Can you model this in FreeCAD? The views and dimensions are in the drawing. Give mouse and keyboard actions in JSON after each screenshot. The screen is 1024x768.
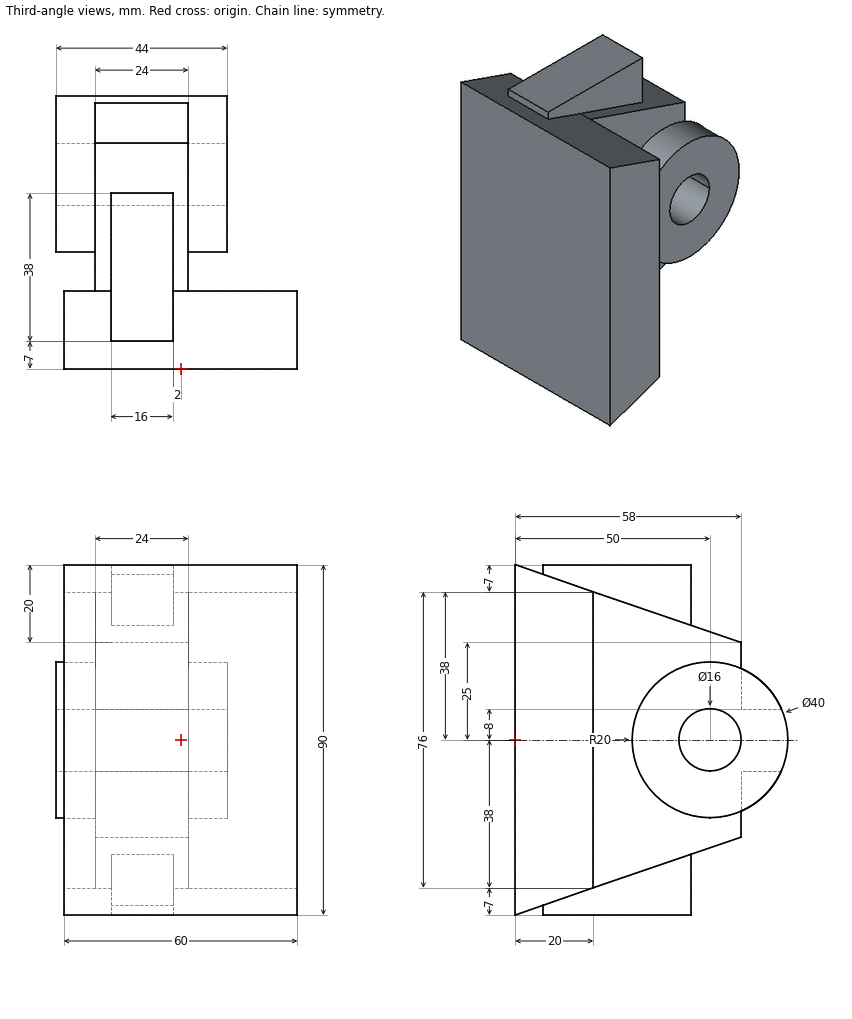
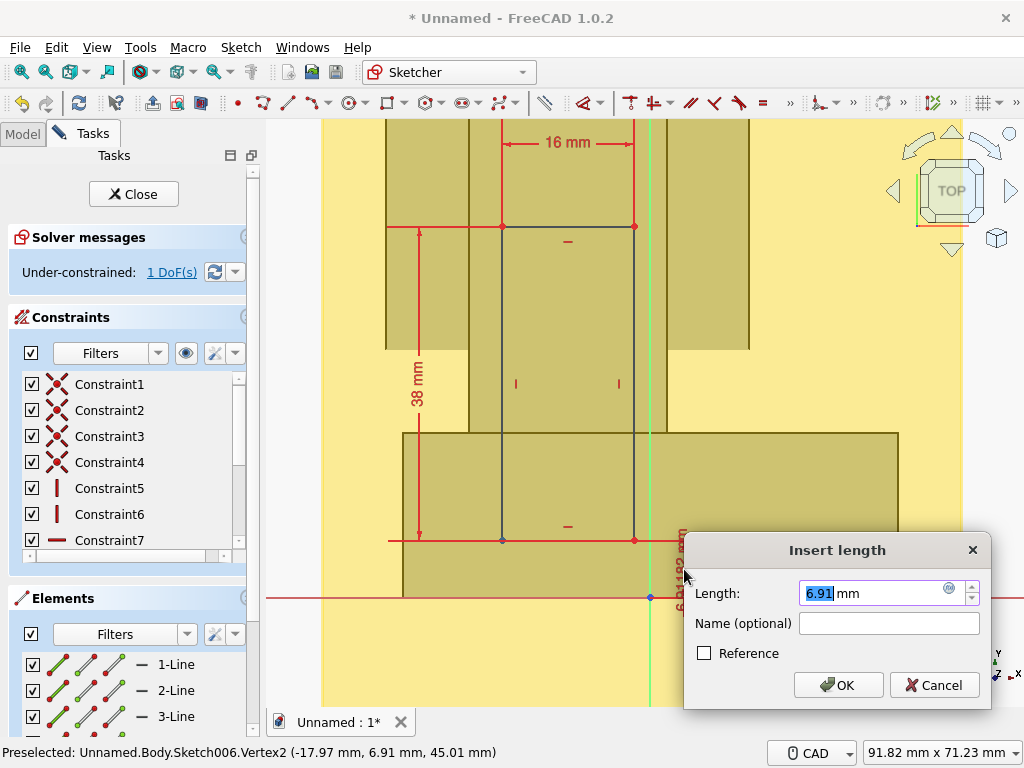
{"action": "type", "text": "7"}
{"action": "key", "text": "Return"}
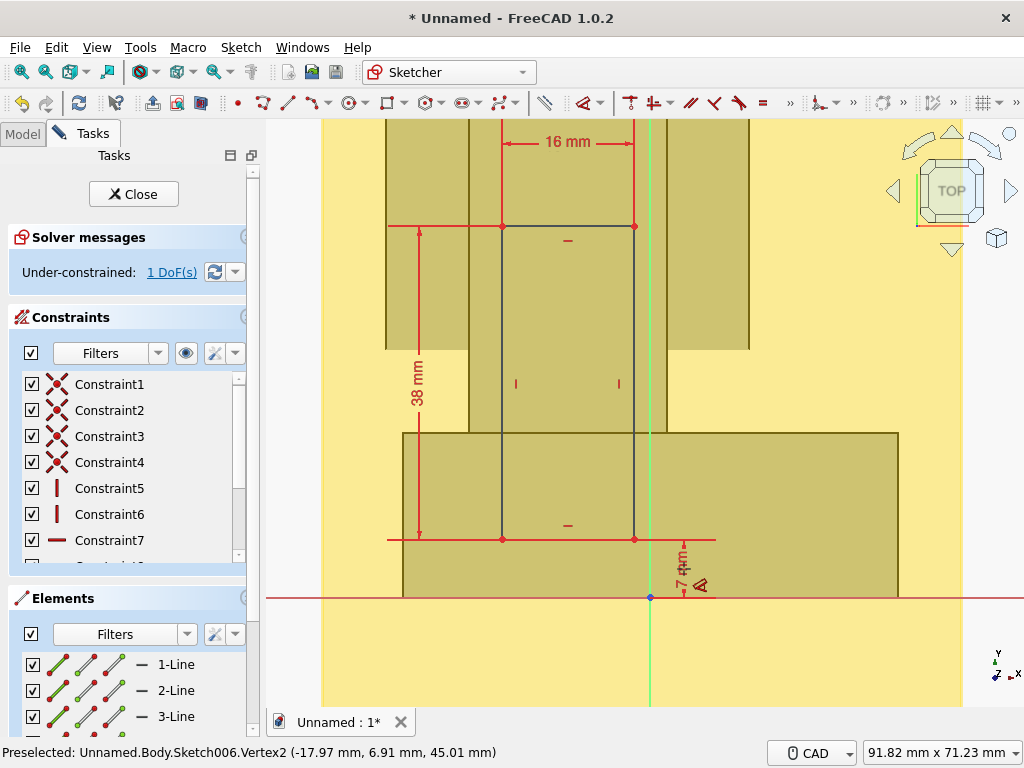
{"action": "scroll", "coordinate": [634, 540], "scroll_direction": "up", "scroll_amount": 5}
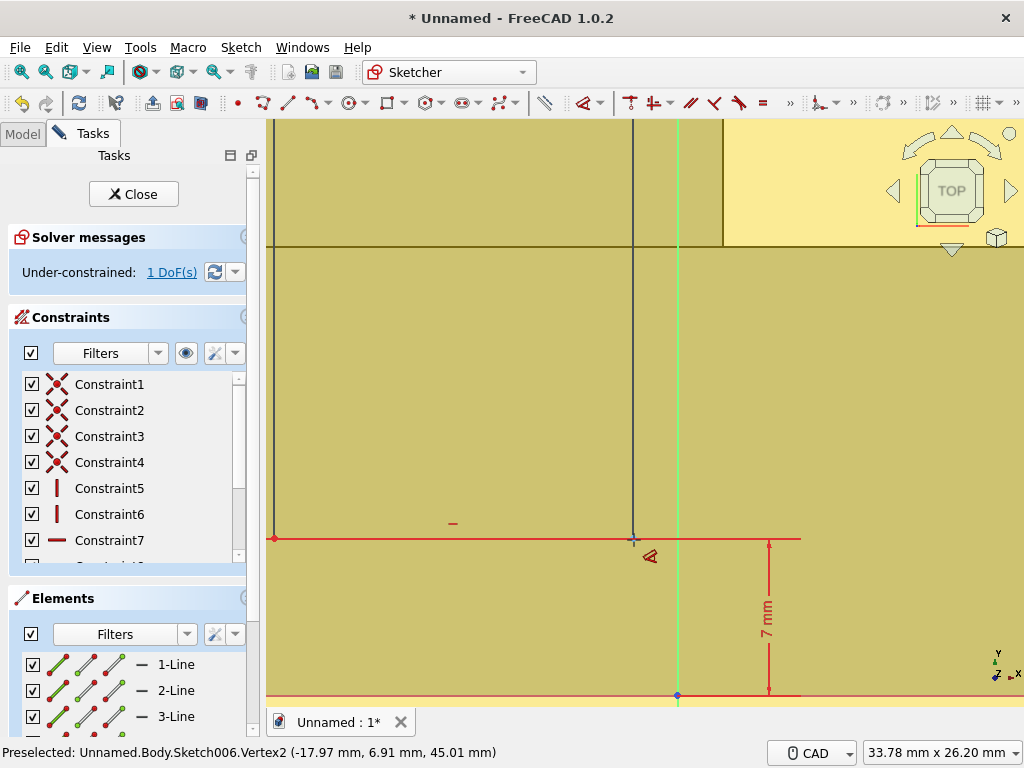
{"action": "left_click", "coordinate": [633, 539]}
{"action": "left_click", "coordinate": [656, 505]}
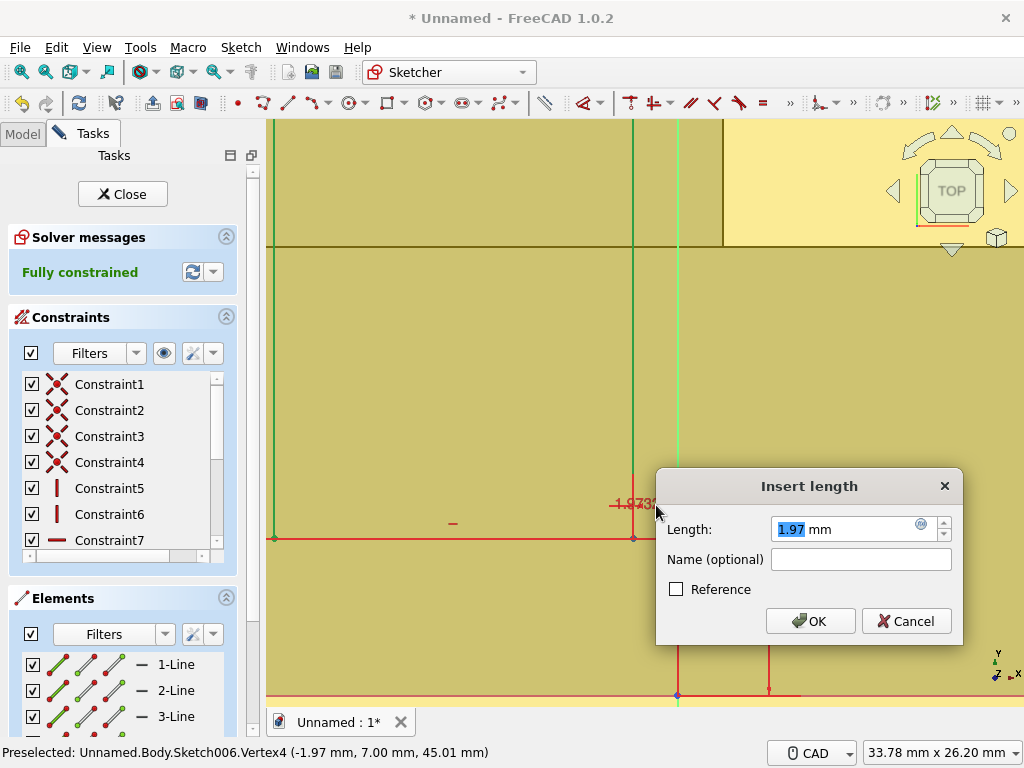
{"action": "type", "text": "2"}
{"action": "key", "text": "Return"}
{"action": "key", "text": "Escape"}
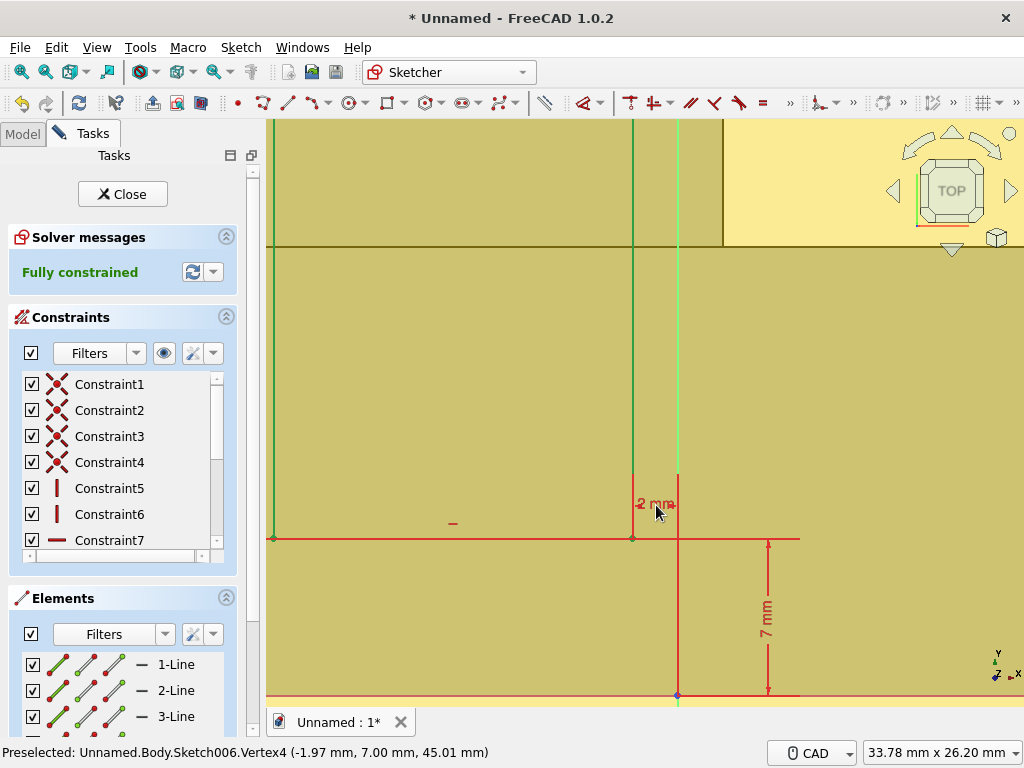
{"action": "left_click", "coordinate": [123, 194]}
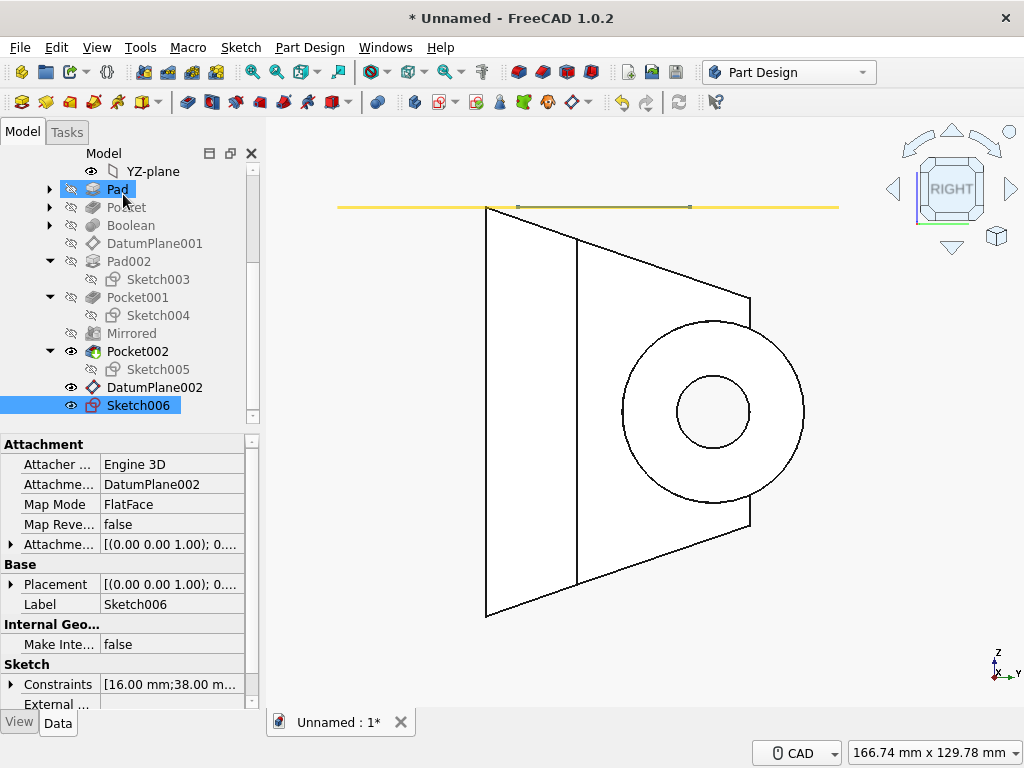
{"action": "left_click", "coordinate": [22, 102]}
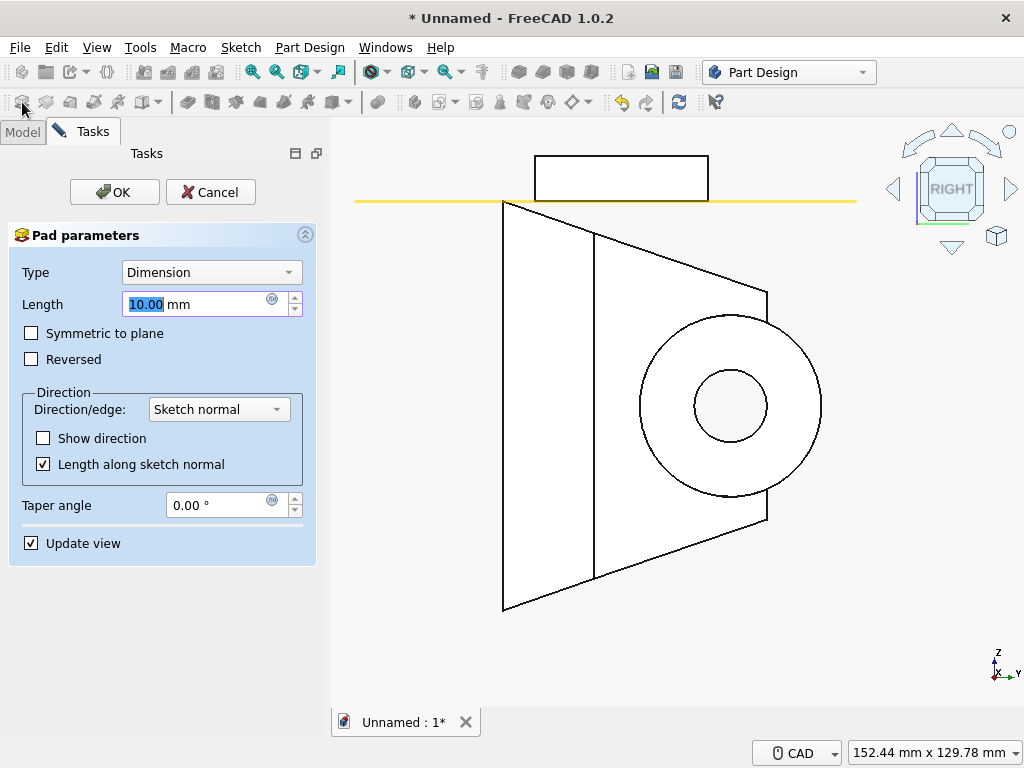
{"action": "type", "text": "20"}
{"action": "key", "text": "Tab"}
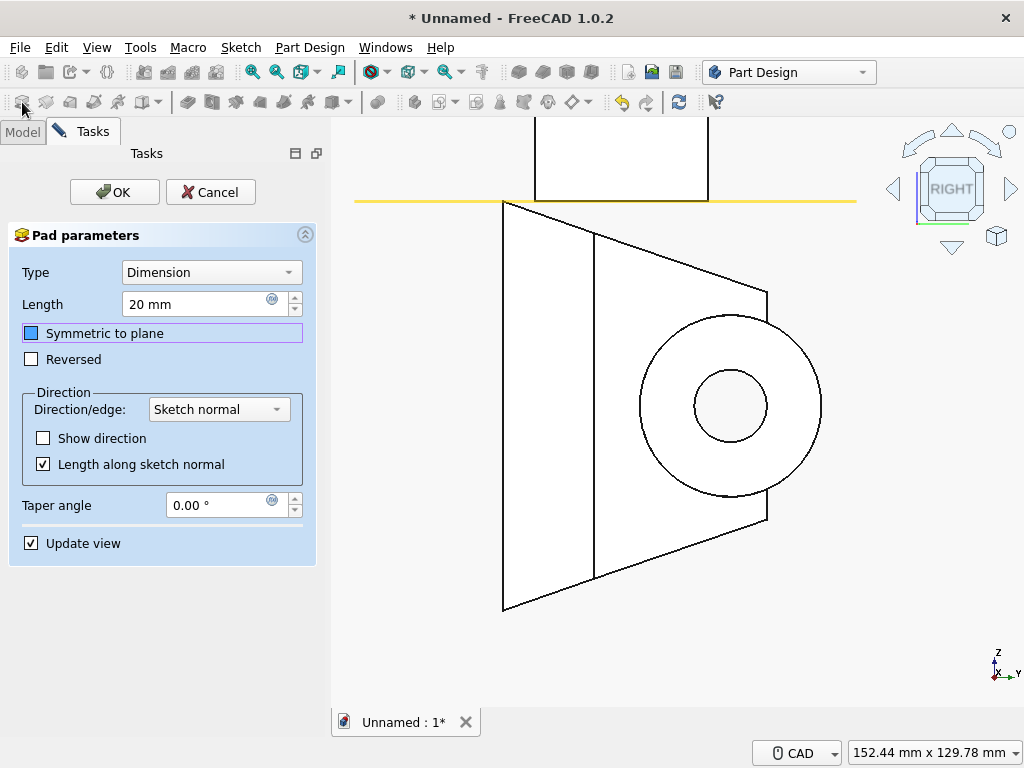
{"action": "left_click", "coordinate": [30, 359]}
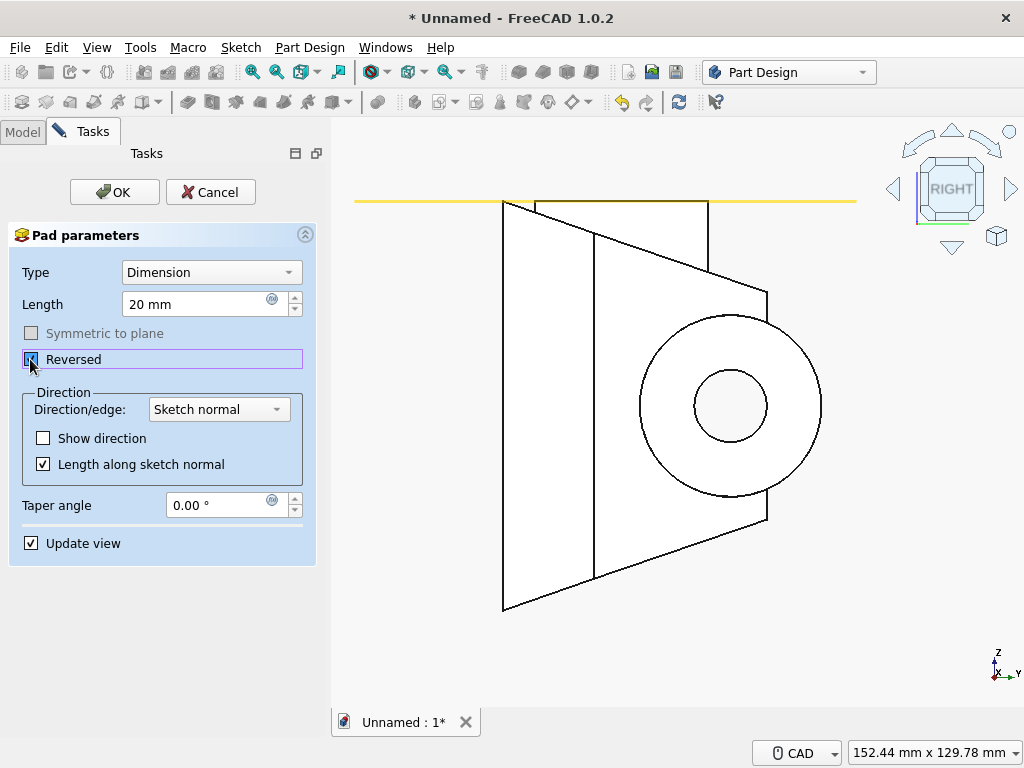
{"action": "left_click", "coordinate": [115, 192]}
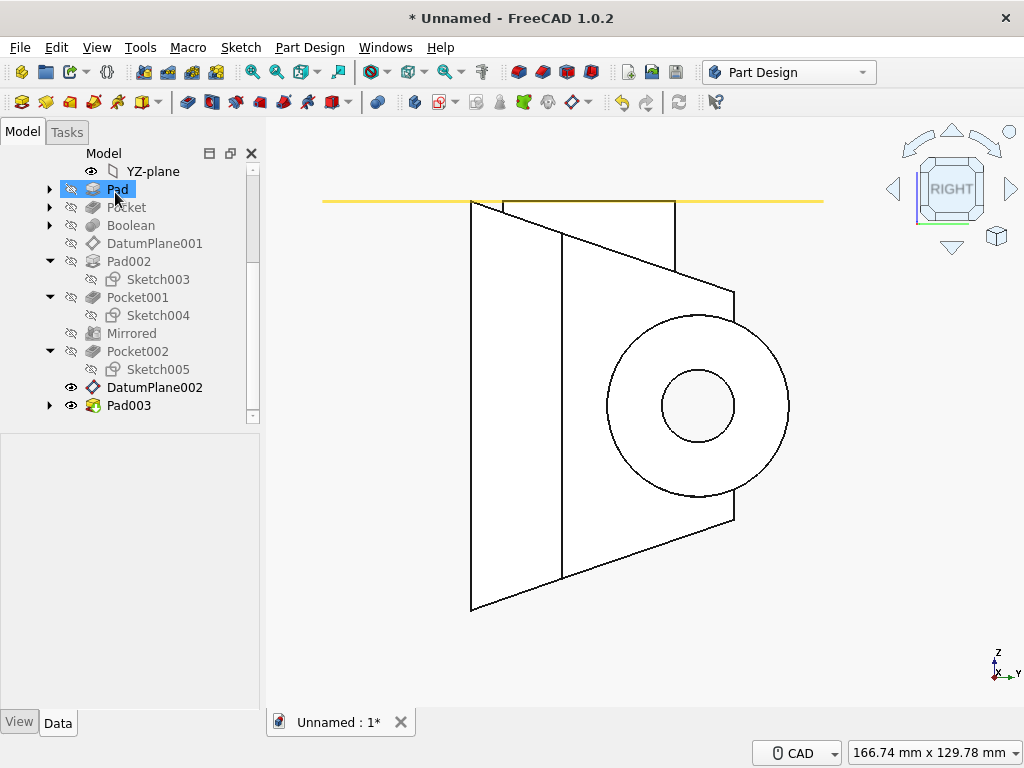
{"action": "left_click", "coordinate": [116, 387]}
{"action": "key", "text": "space"}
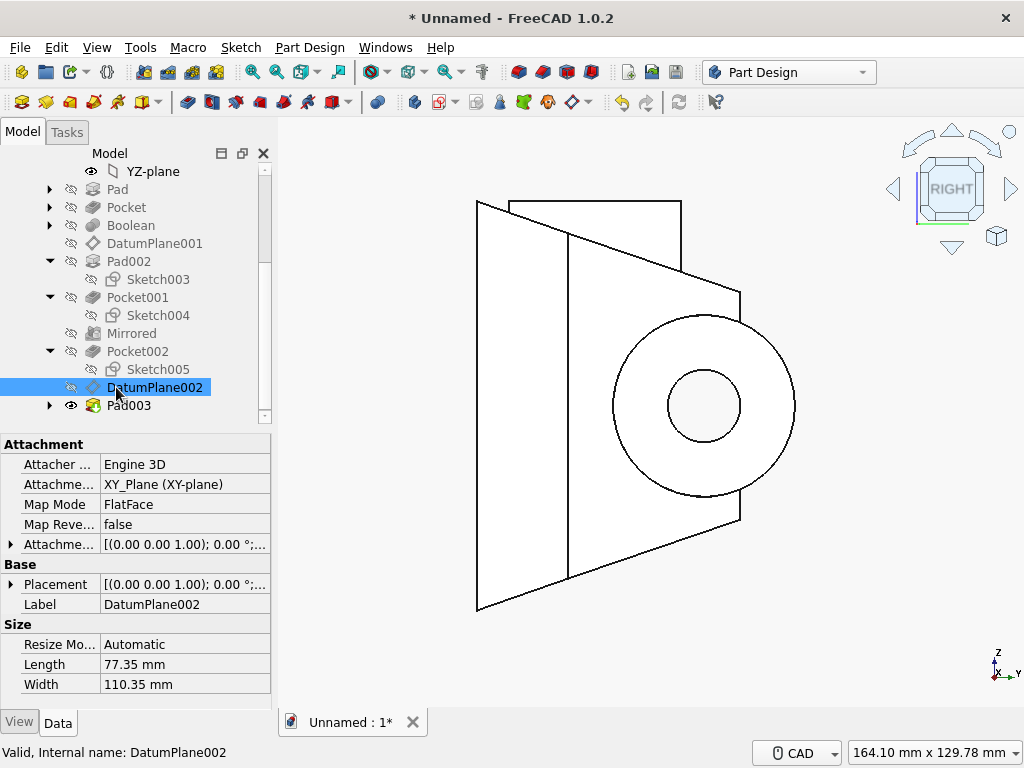
{"action": "left_click", "coordinate": [116, 405]}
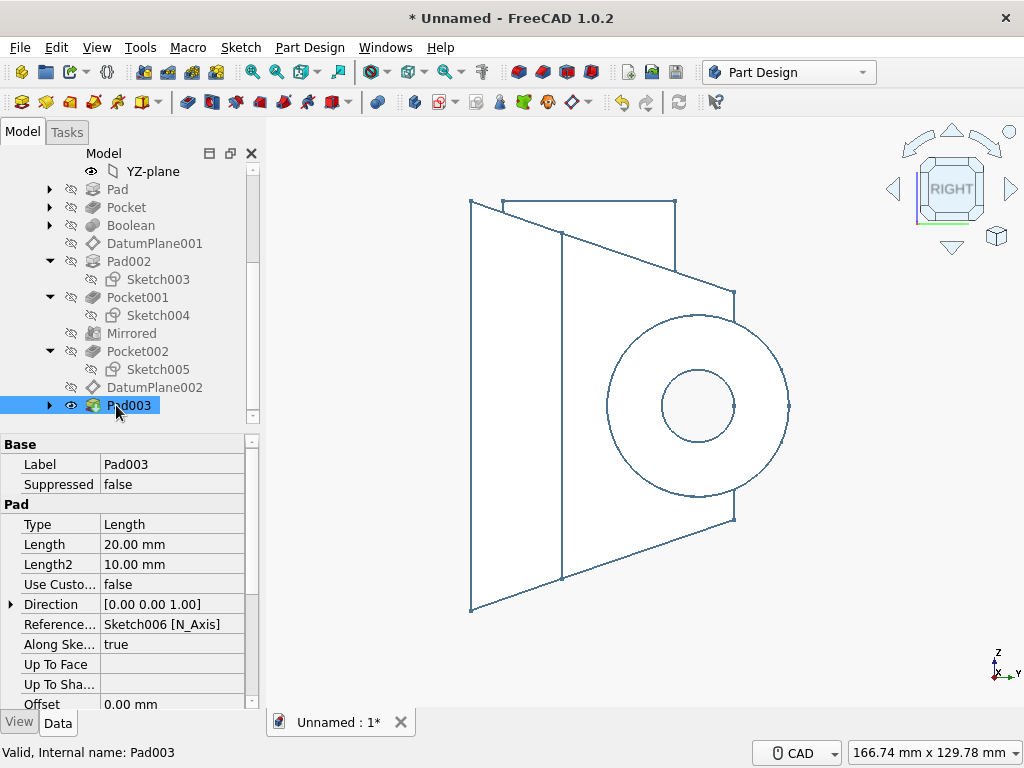
{"action": "left_click", "coordinate": [144, 72]}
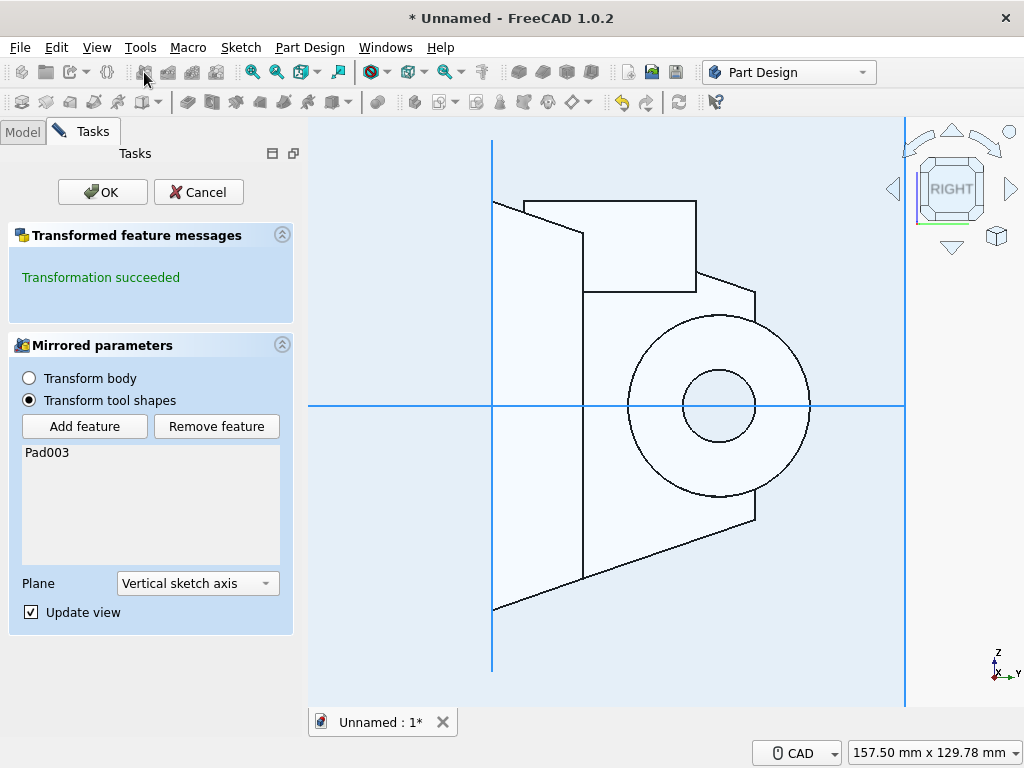
{"action": "left_click", "coordinate": [198, 584]}